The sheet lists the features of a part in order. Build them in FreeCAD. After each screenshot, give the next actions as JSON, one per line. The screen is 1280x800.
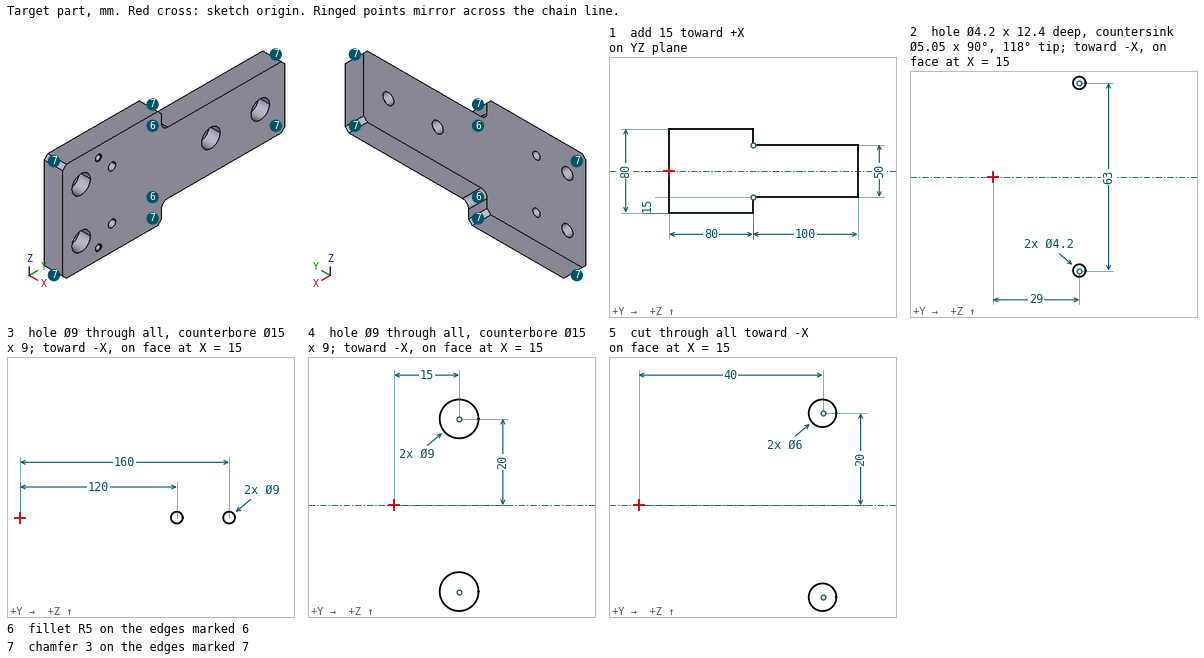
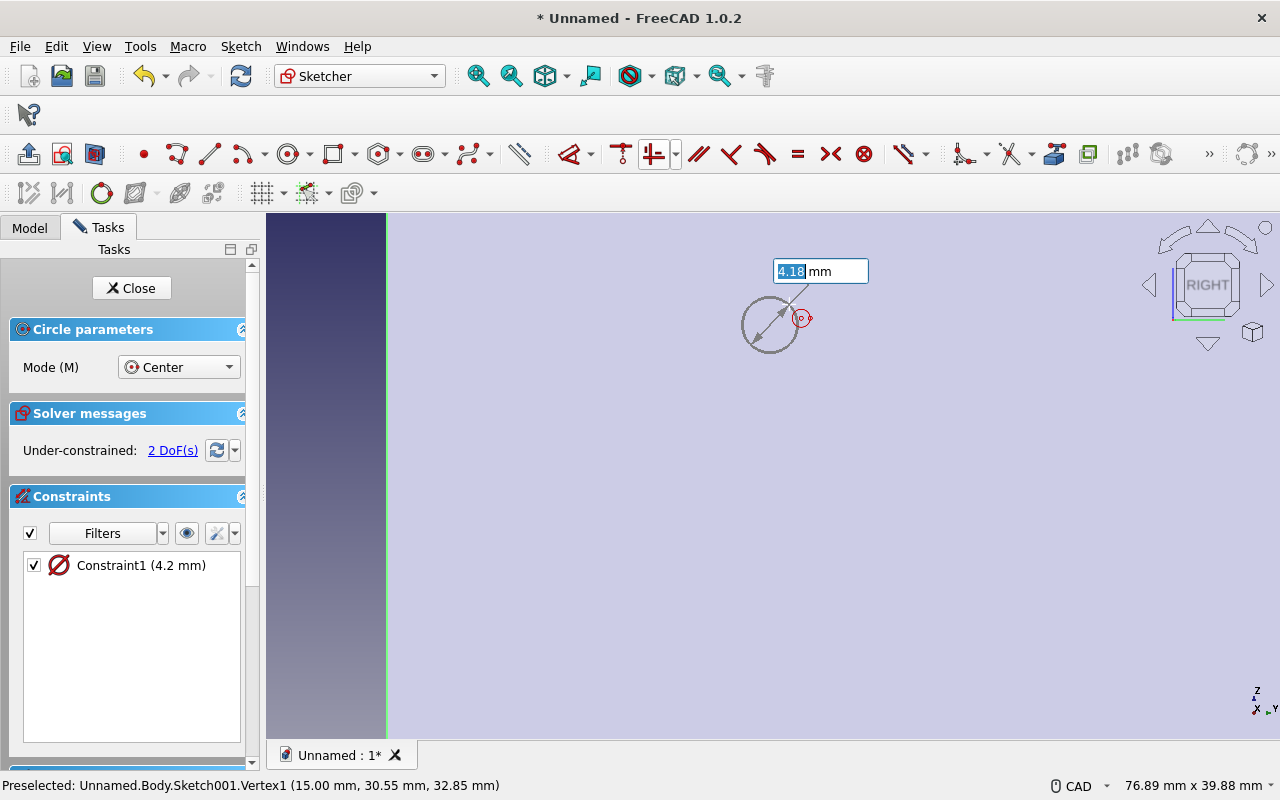
{"action": "type", "text": "4.2"}
{"action": "key", "text": "Return"}
{"action": "key", "text": "Escape"}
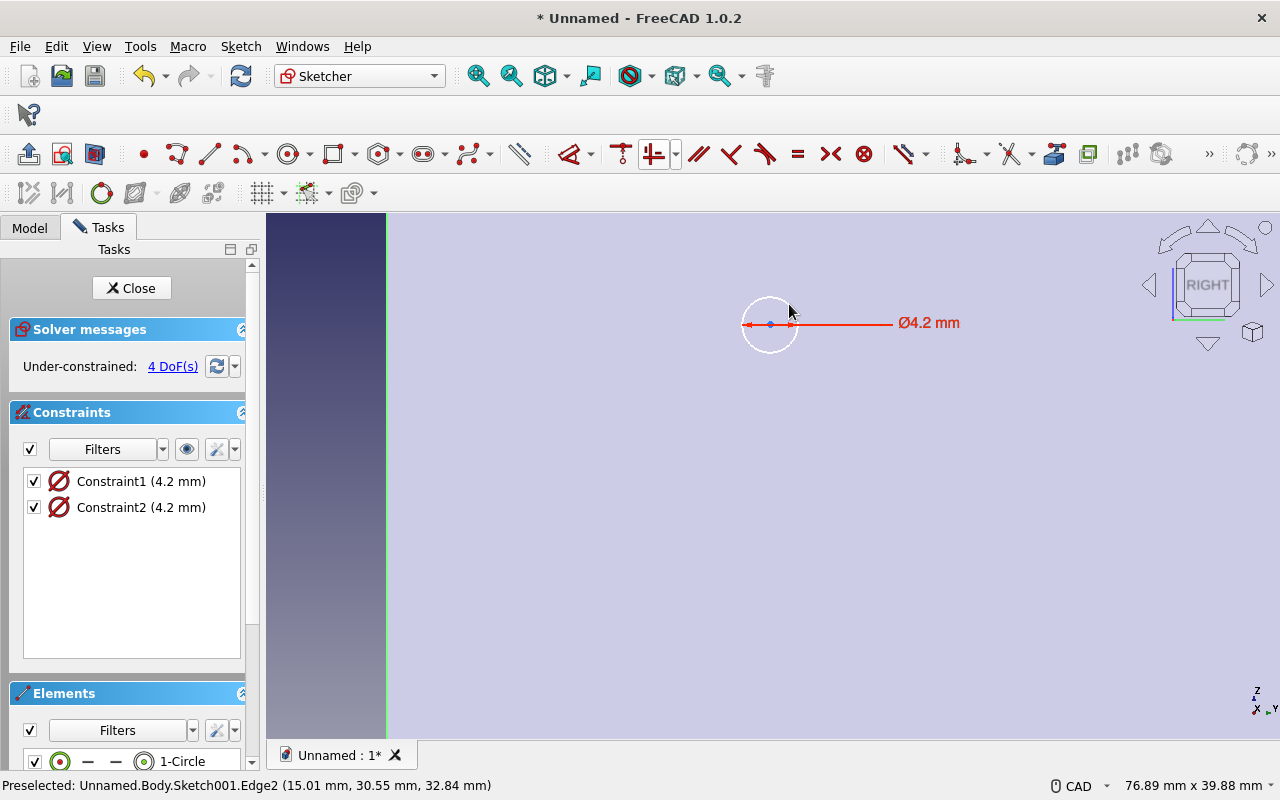
{"action": "scroll", "coordinate": [770, 323], "scroll_direction": "down", "scroll_amount": 5}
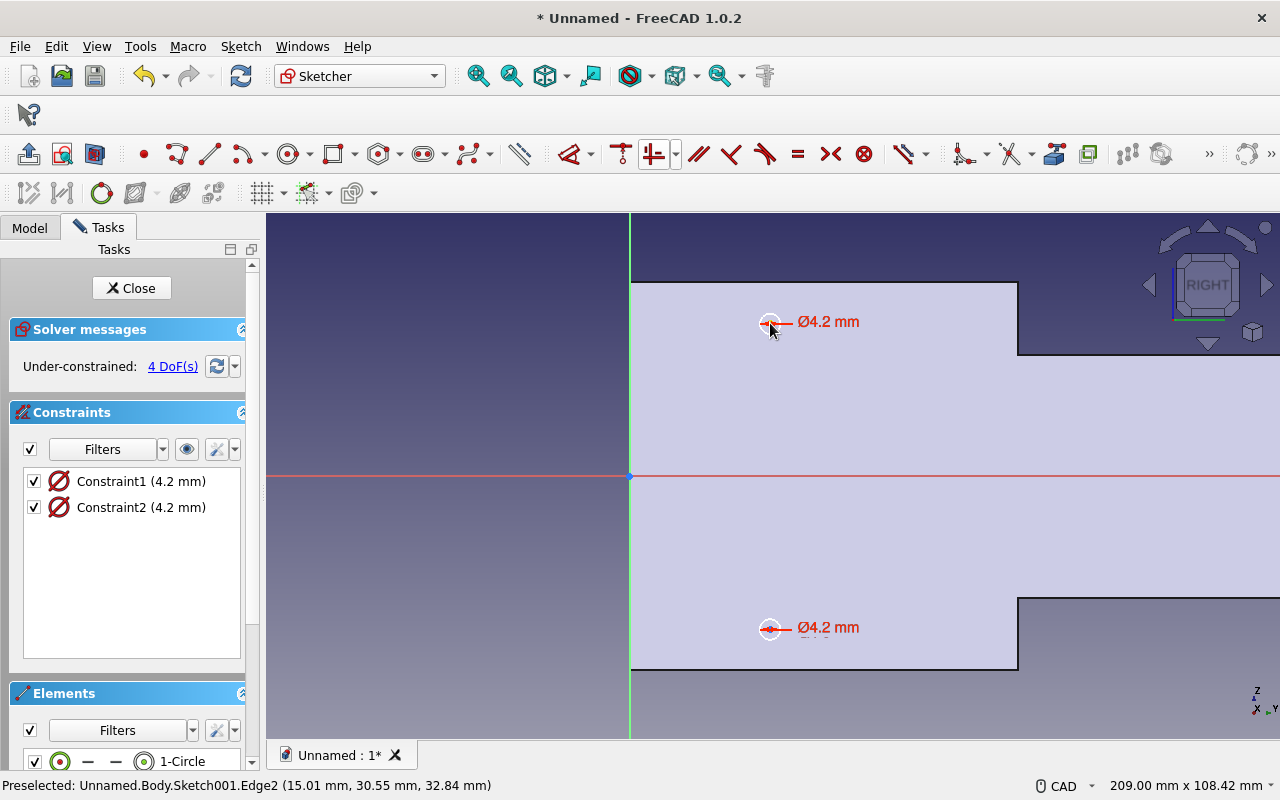
{"action": "left_click", "coordinate": [770, 630]}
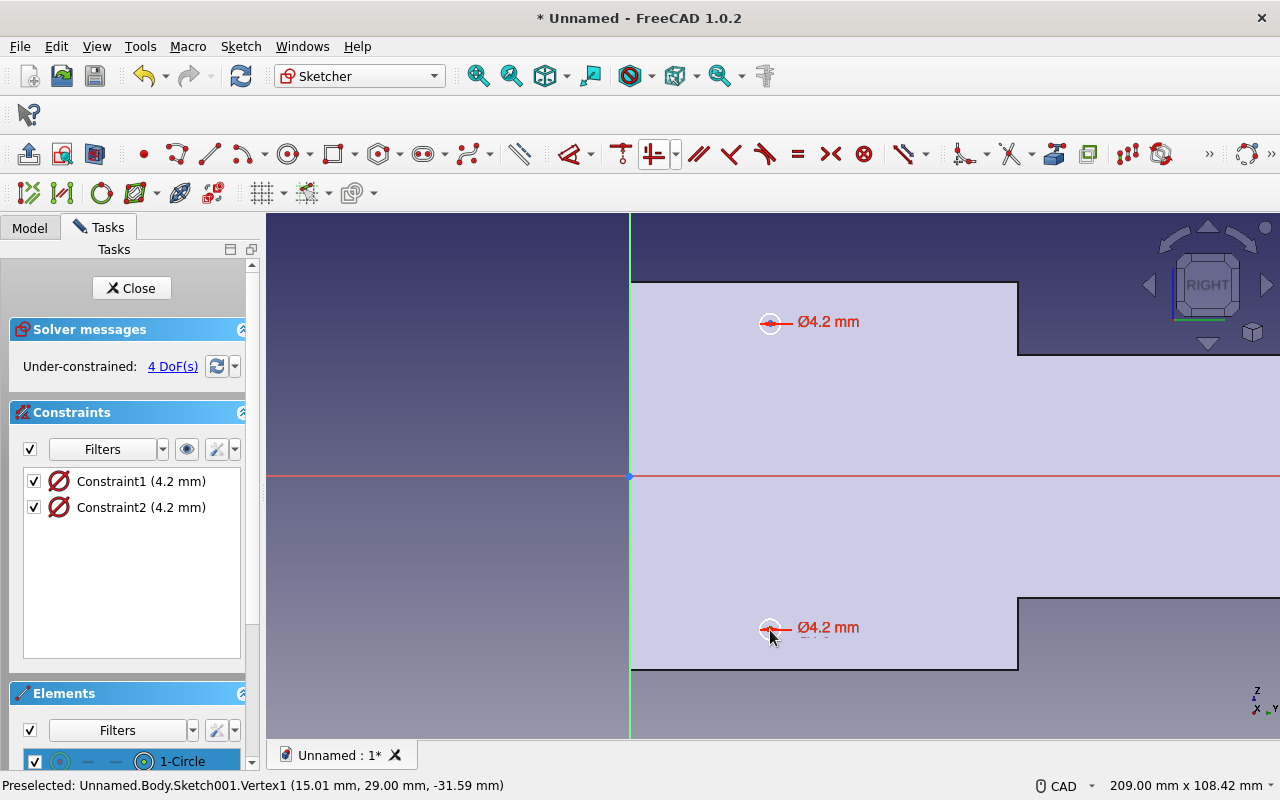
{"action": "left_click", "coordinate": [770, 324]}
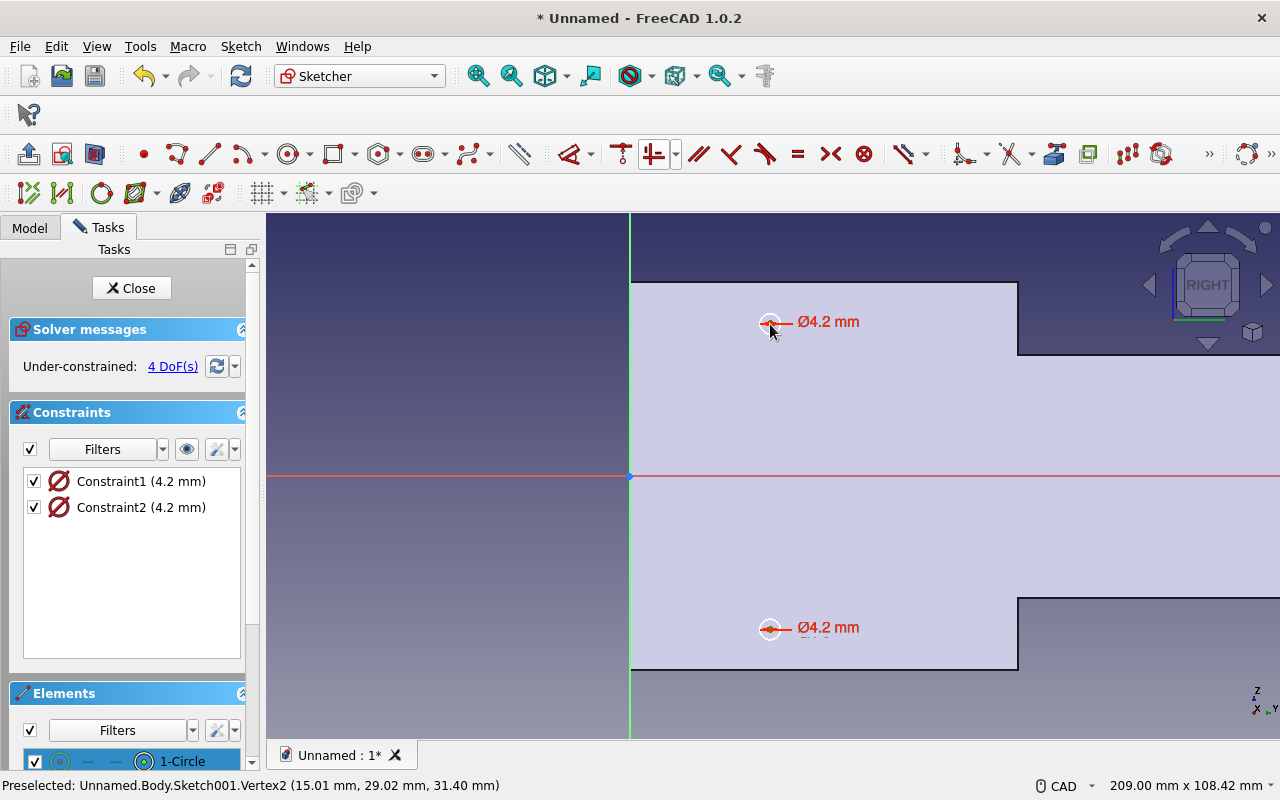
{"action": "left_click", "coordinate": [353, 476]}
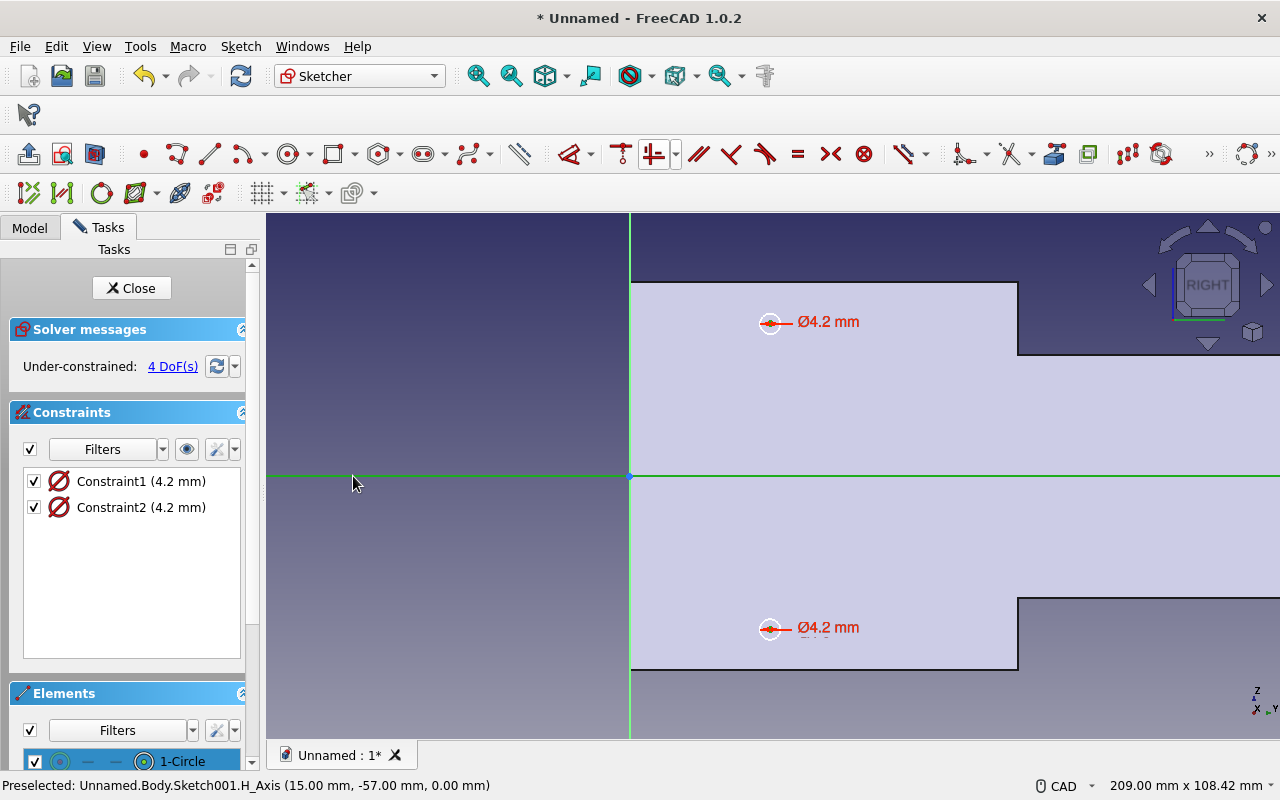
{"action": "left_click", "coordinate": [831, 154]}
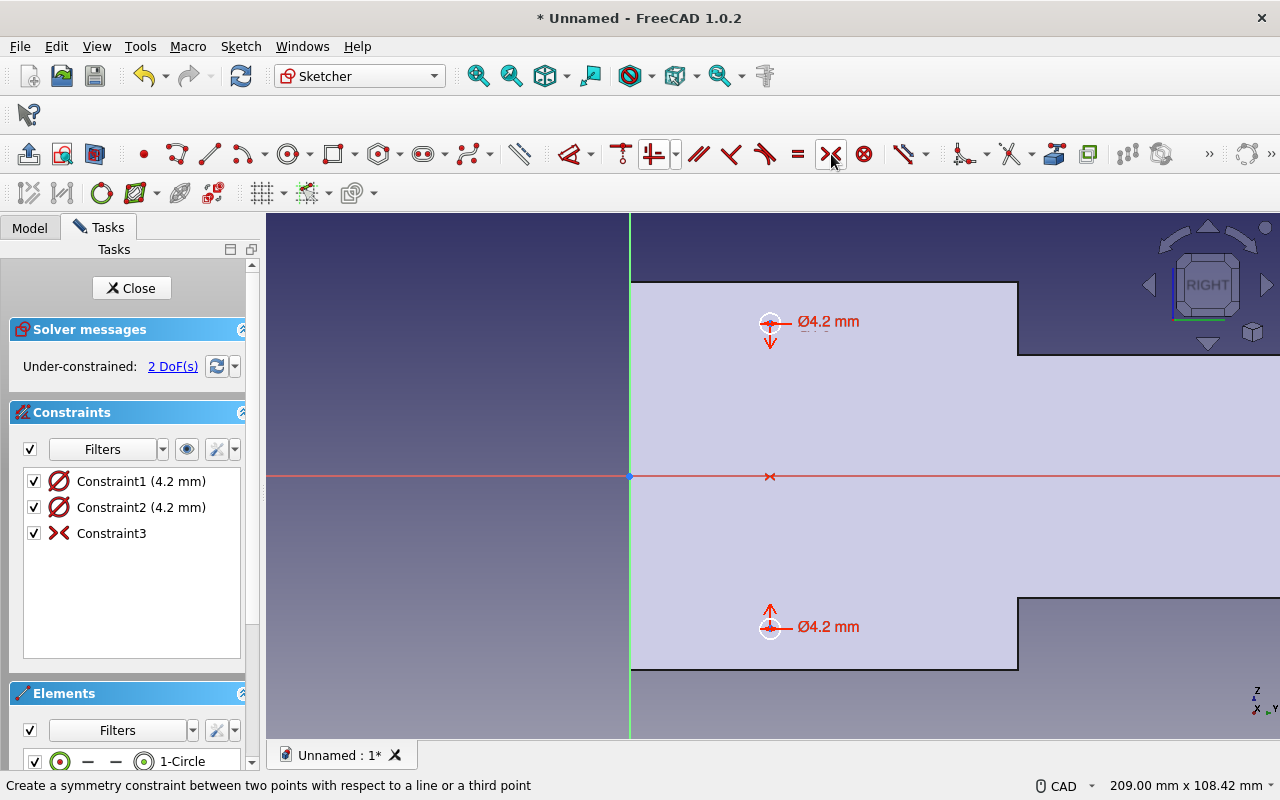
{"action": "left_click", "coordinate": [568, 154]}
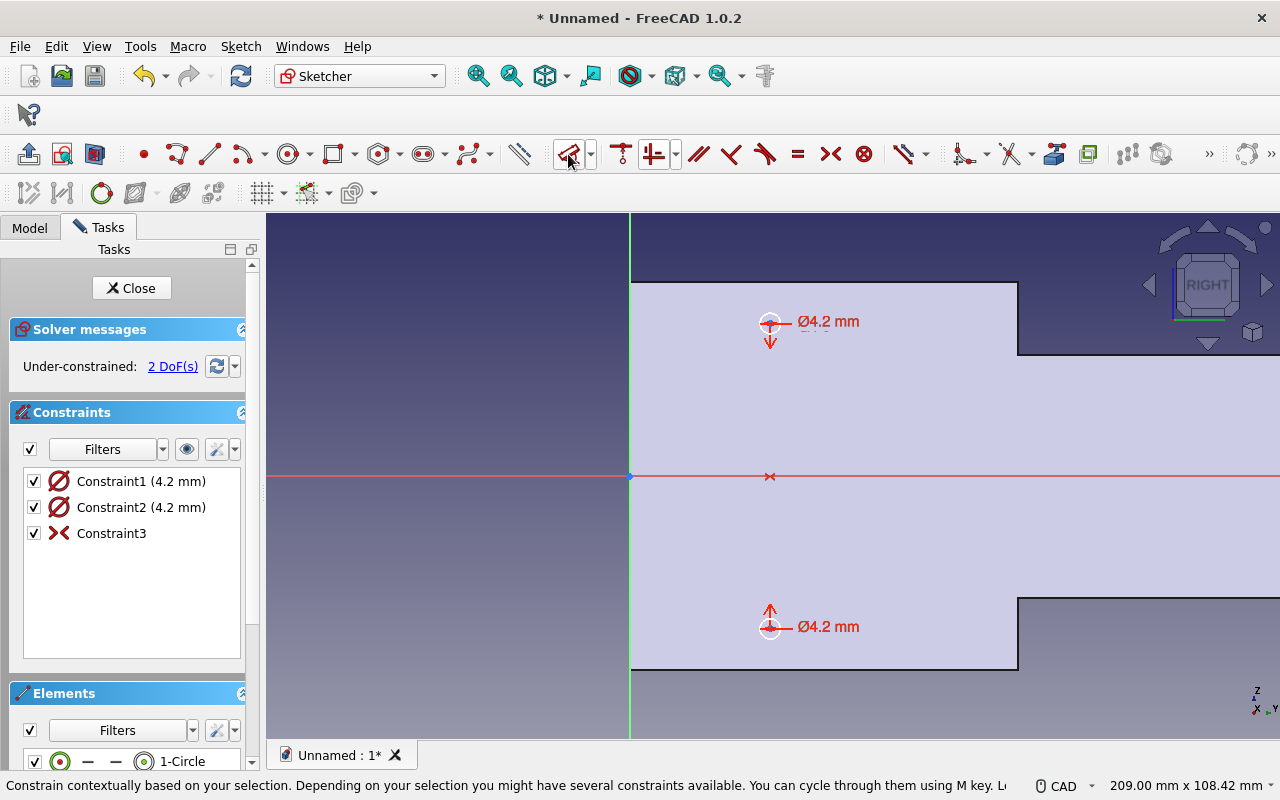
{"action": "left_click", "coordinate": [770, 629]}
{"action": "left_click", "coordinate": [700, 663]}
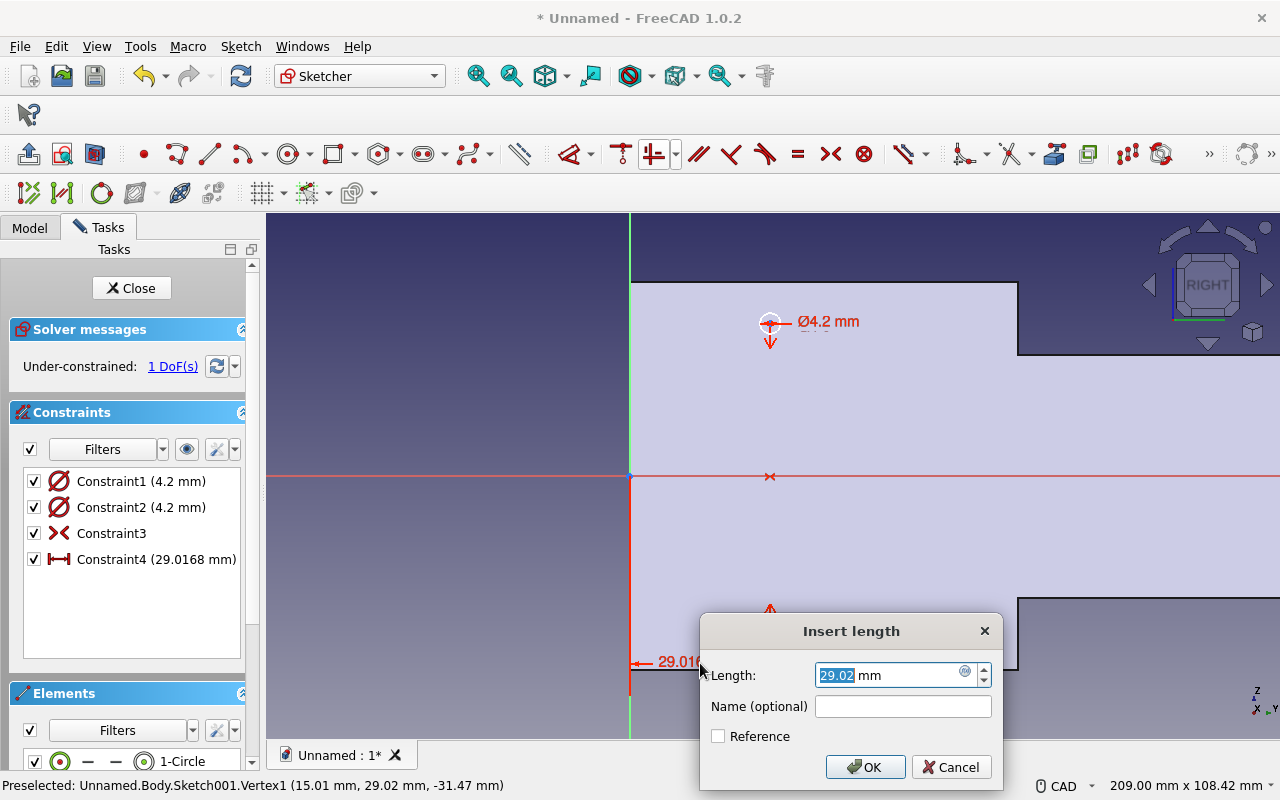
{"action": "type", "text": "29"}
{"action": "key", "text": "Return"}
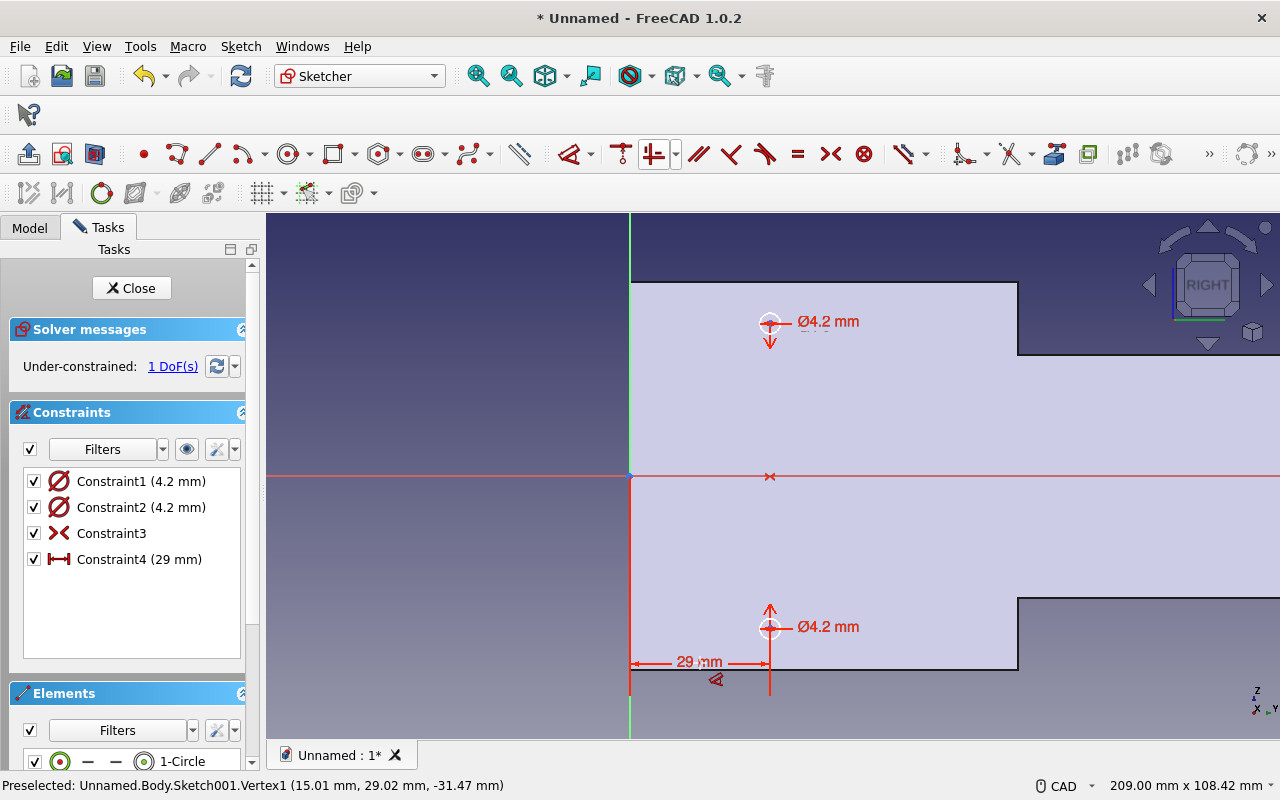
{"action": "left_click", "coordinate": [770, 629]}